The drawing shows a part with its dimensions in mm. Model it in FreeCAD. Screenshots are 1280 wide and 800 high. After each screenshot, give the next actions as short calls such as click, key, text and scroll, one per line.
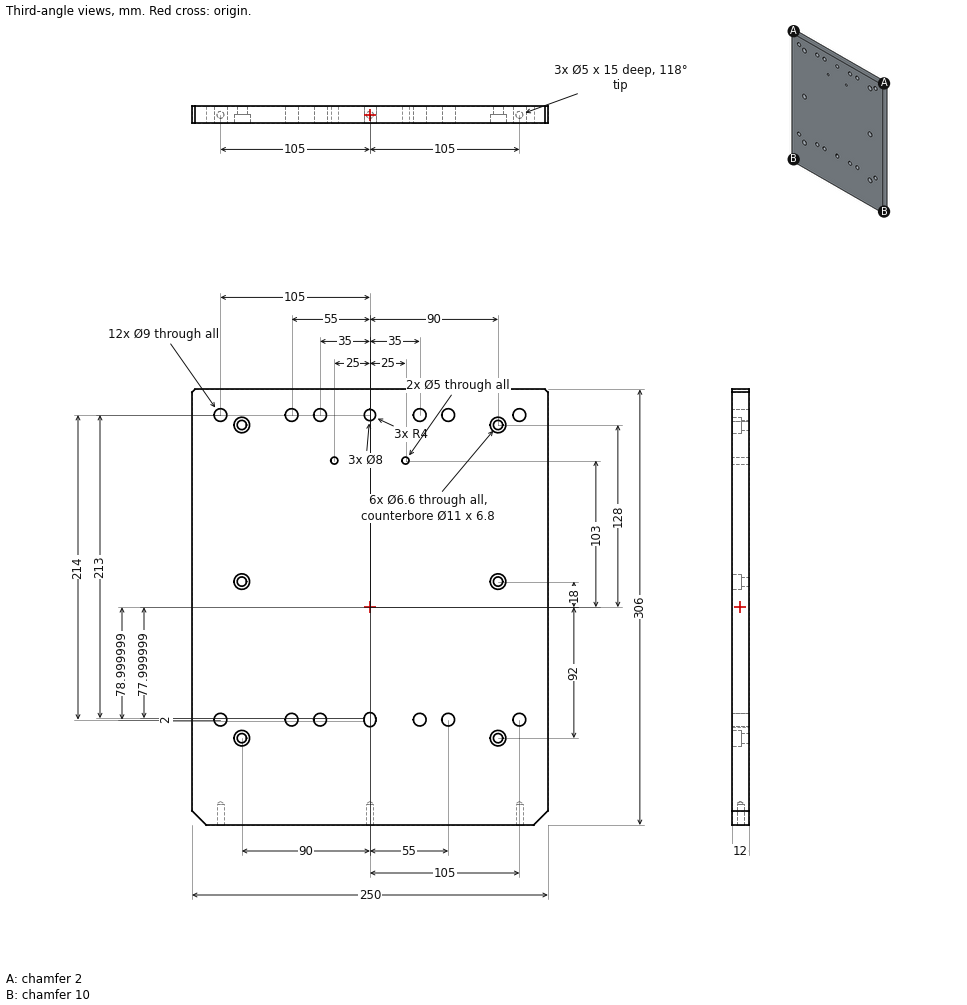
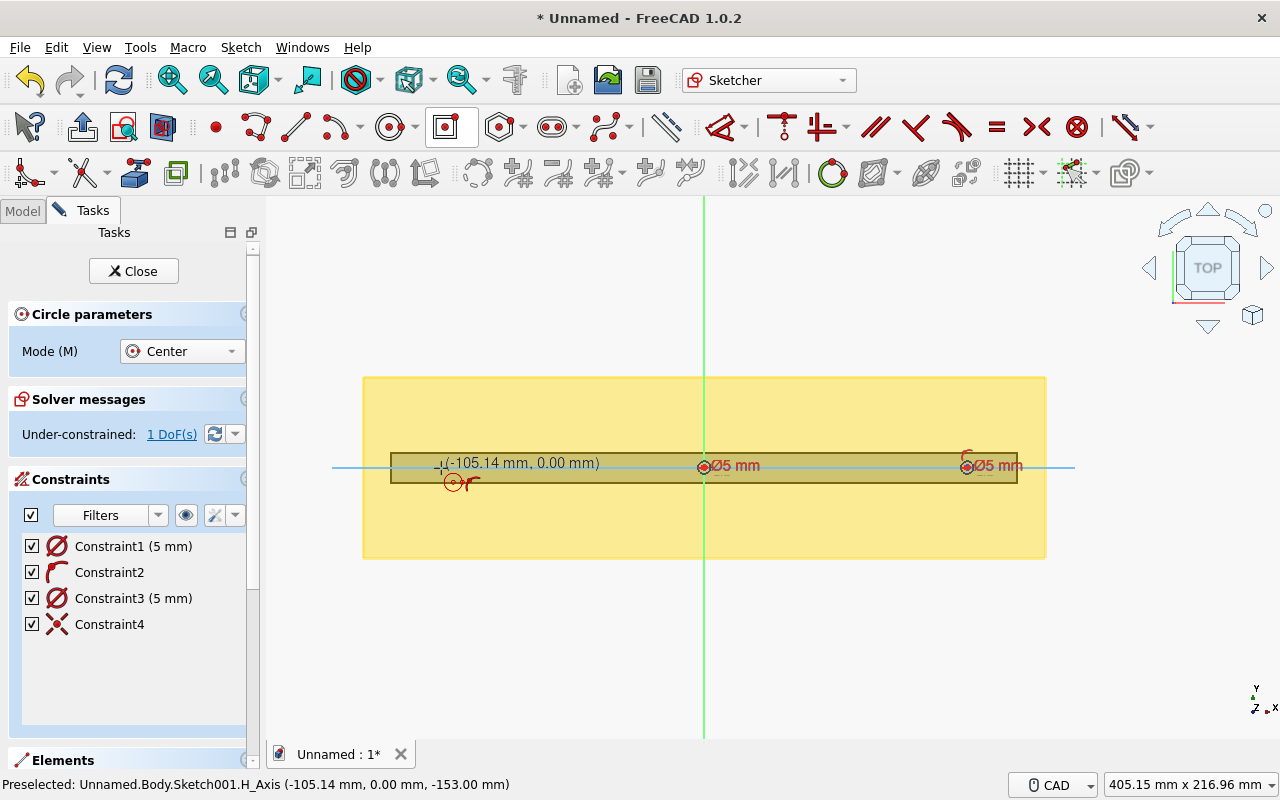
click(441, 468)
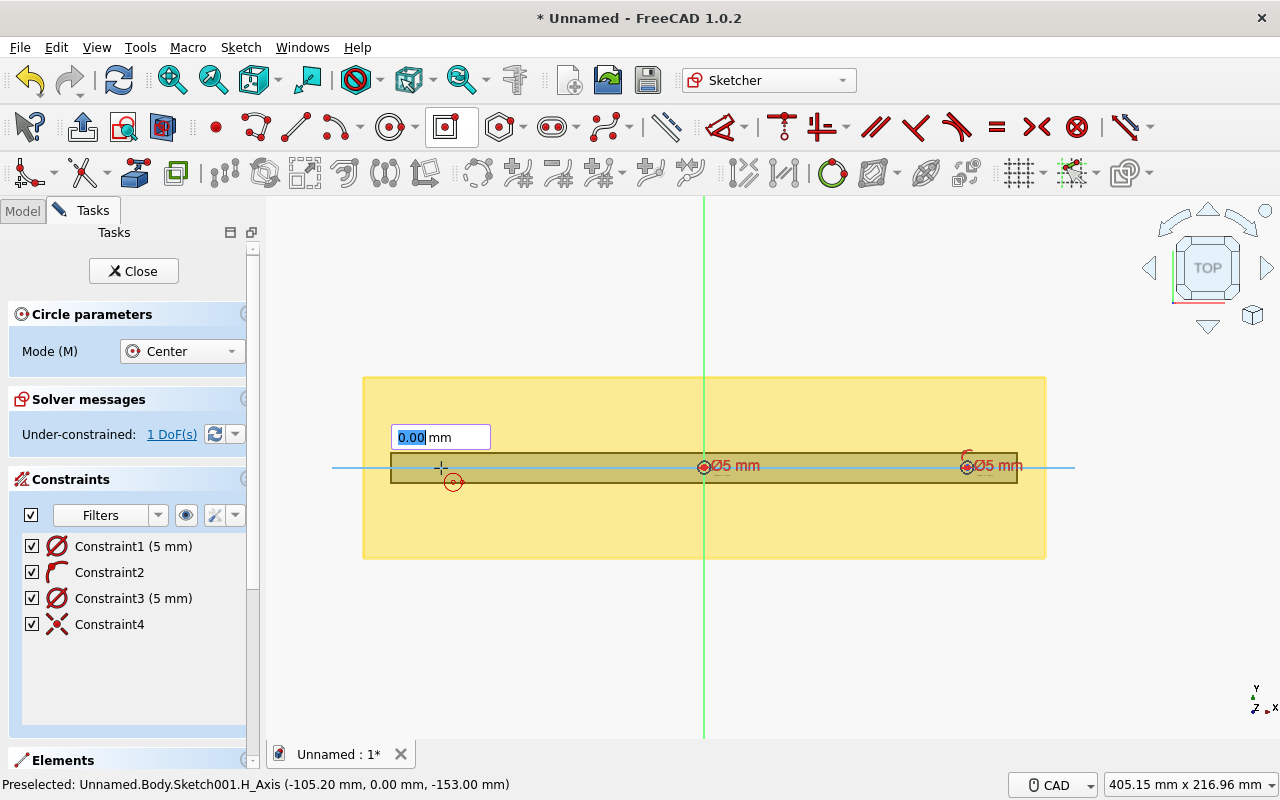
scroll(439, 474, up, 5)
move(440, 472)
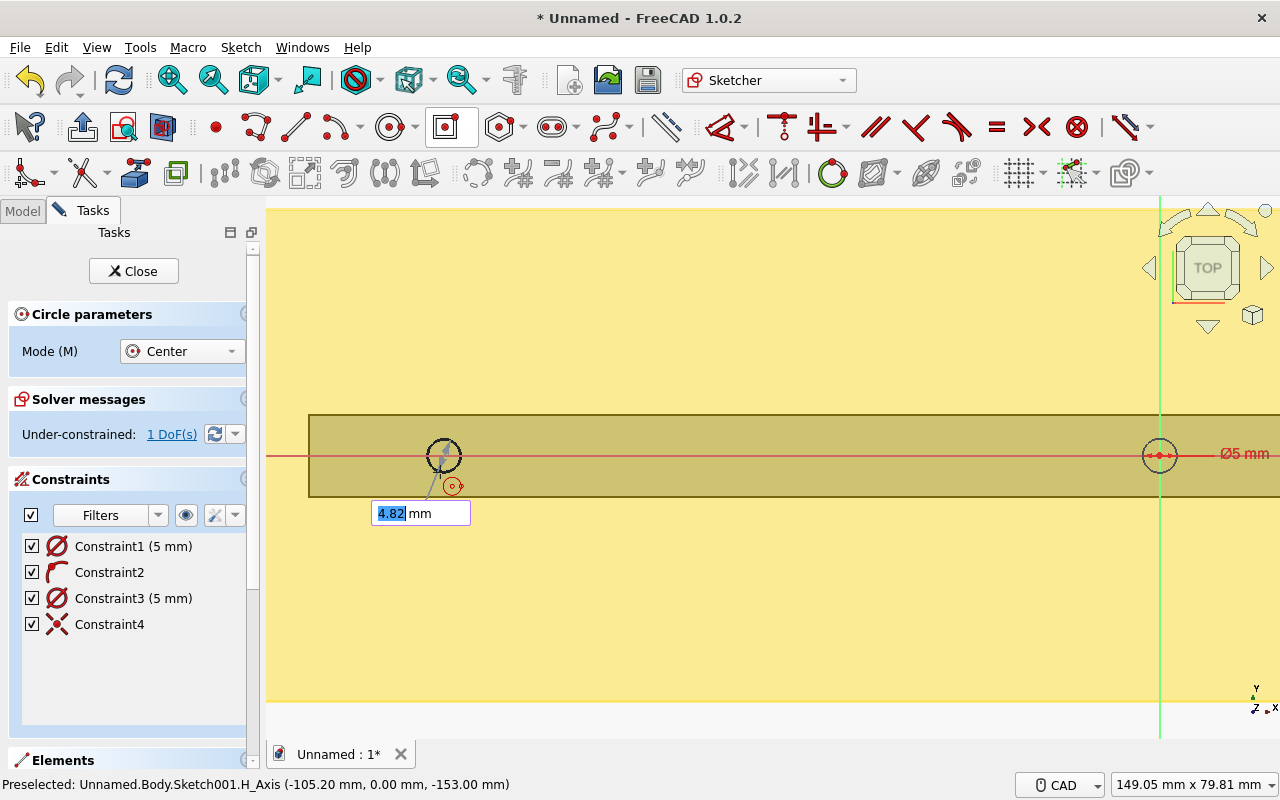
text(5)
key(Return)
key(Escape)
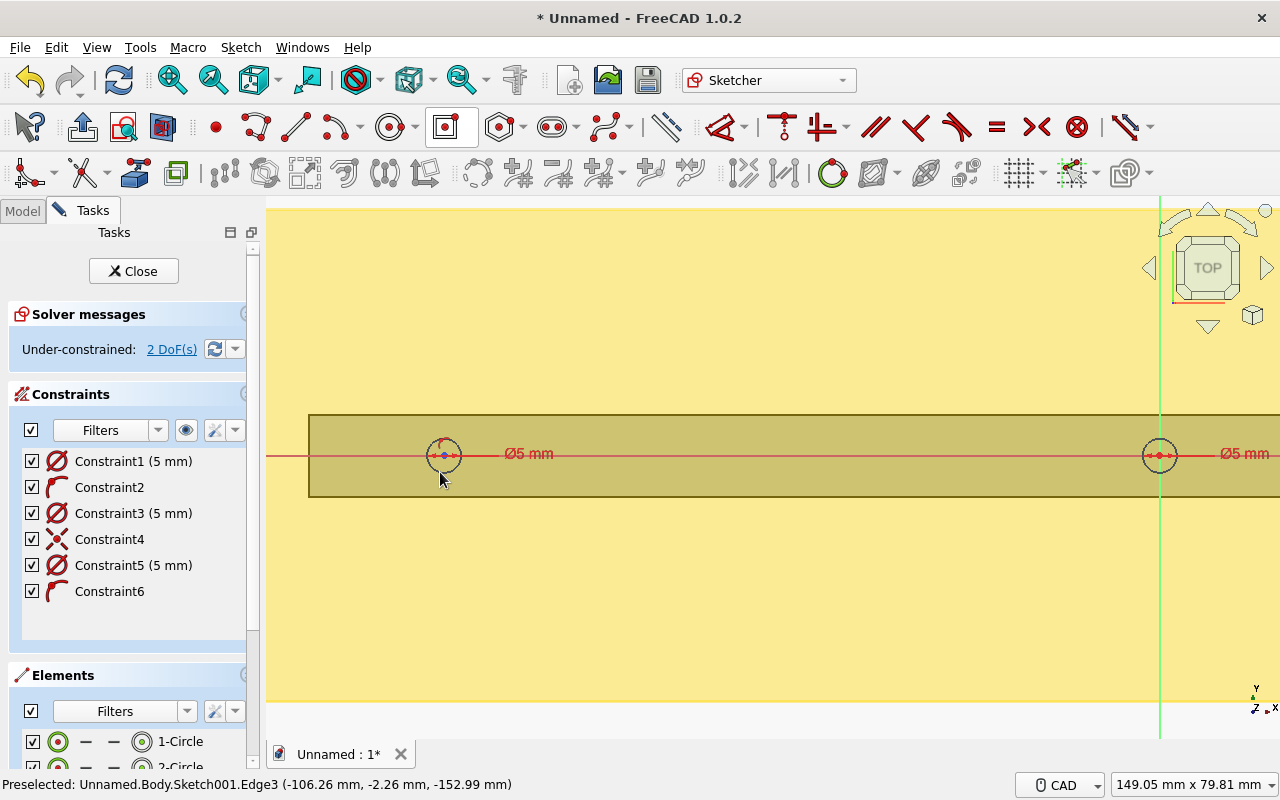
click(720, 128)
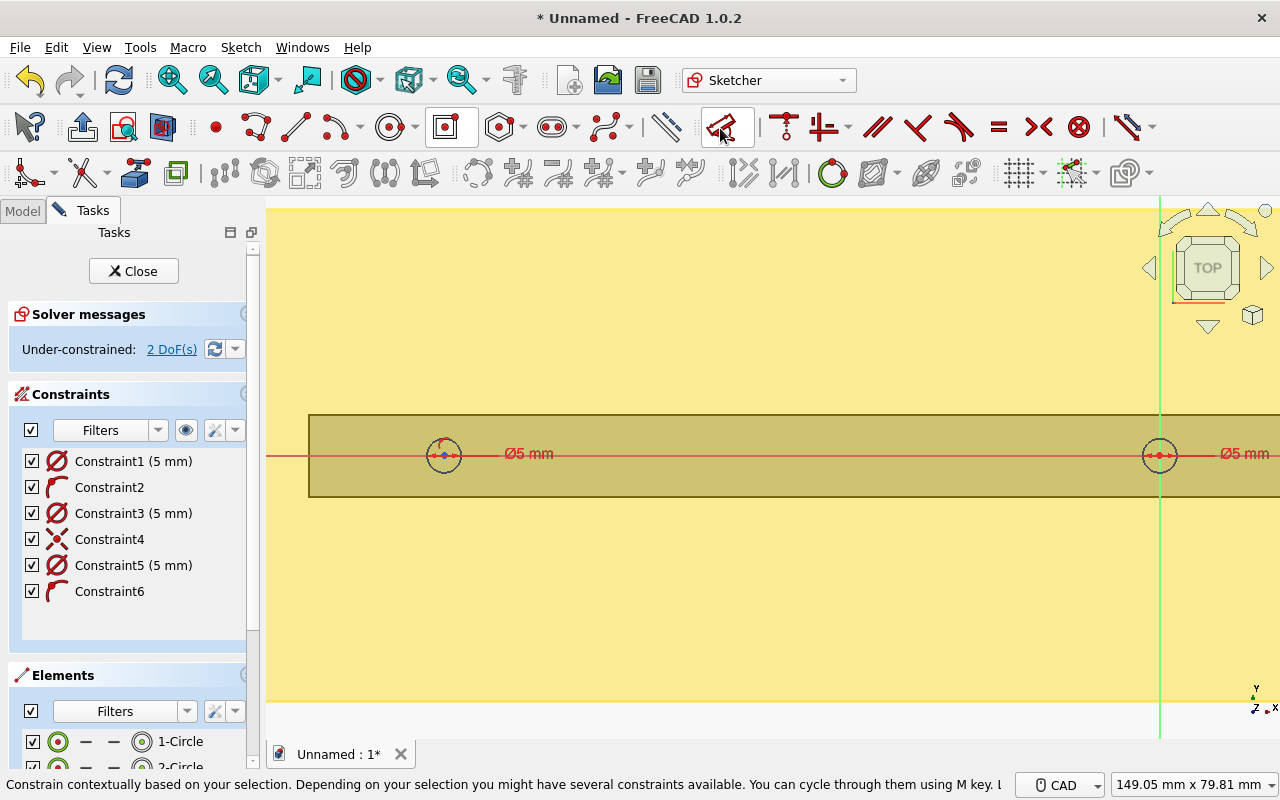
scroll(440, 474, down, 5)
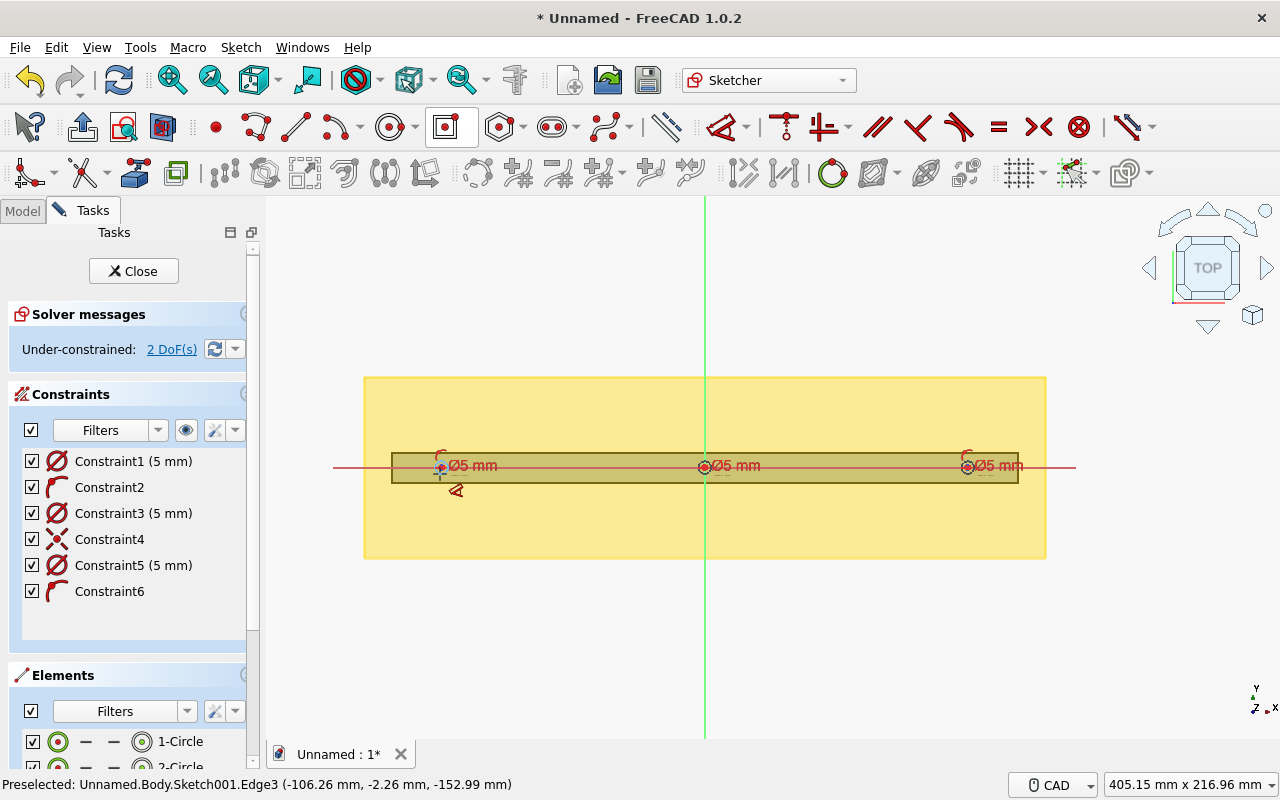
click(968, 468)
click(836, 502)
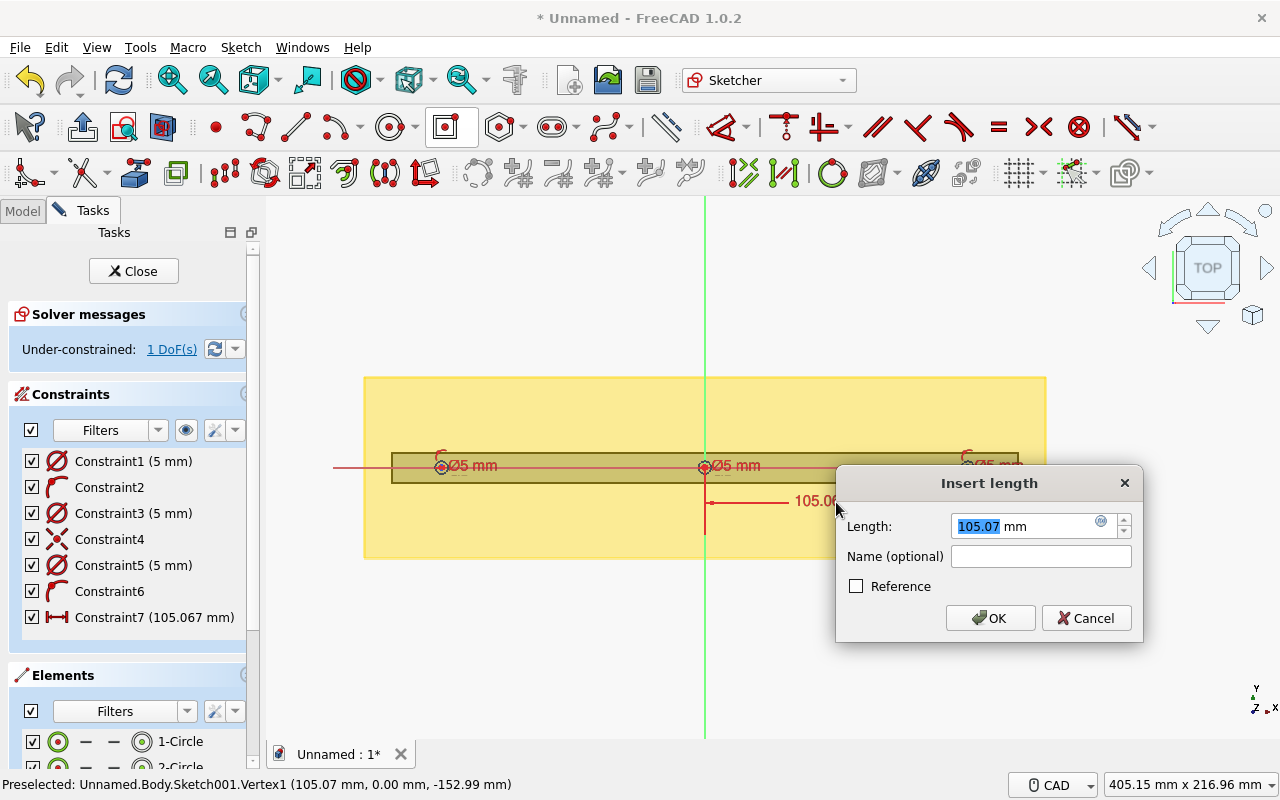
text(105)
key(Return)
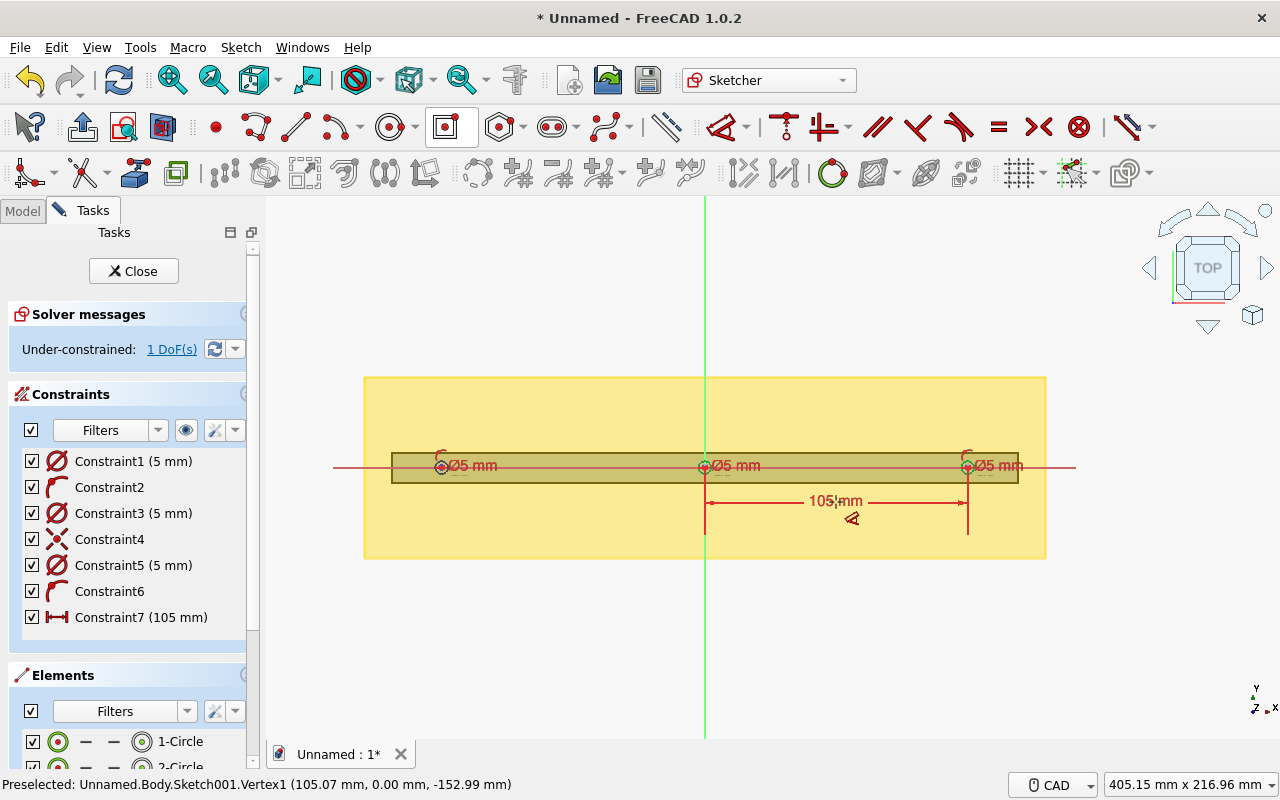
click(442, 468)
click(573, 502)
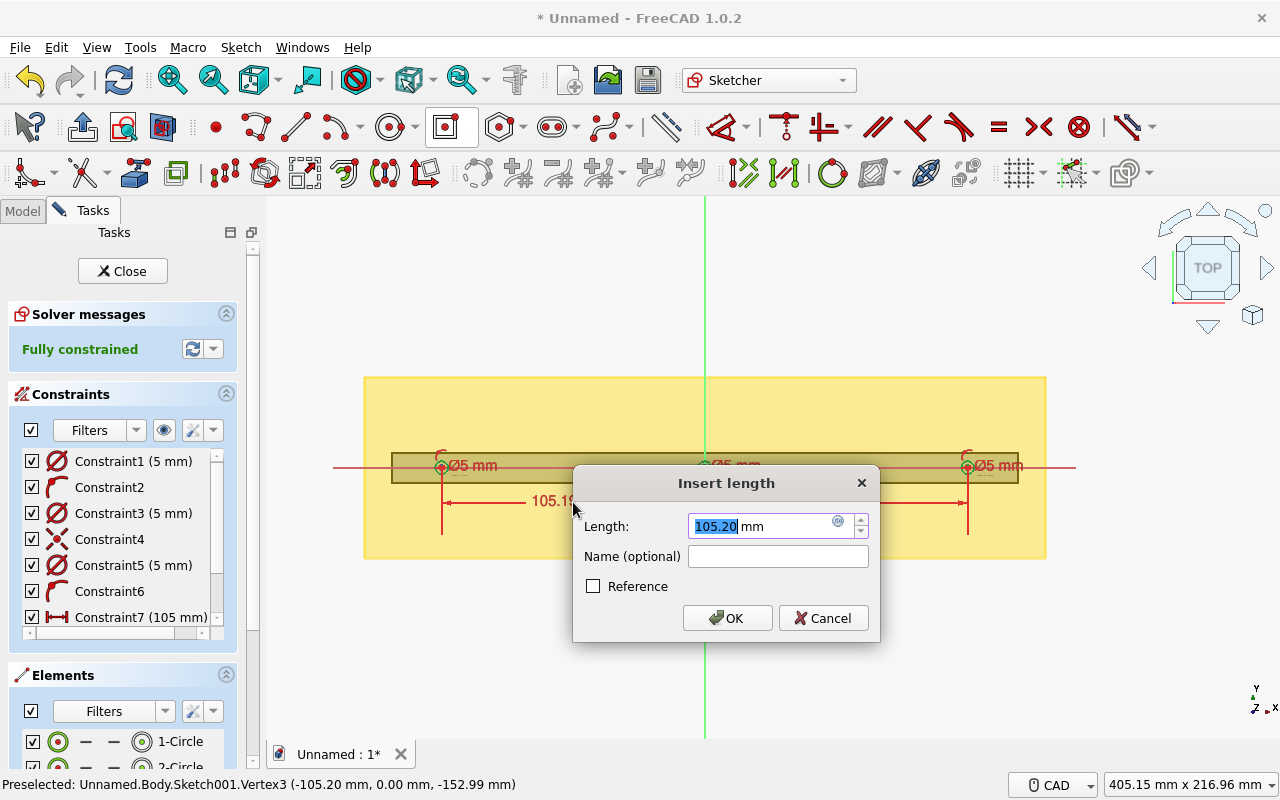
text(105)
key(Return)
key(Escape)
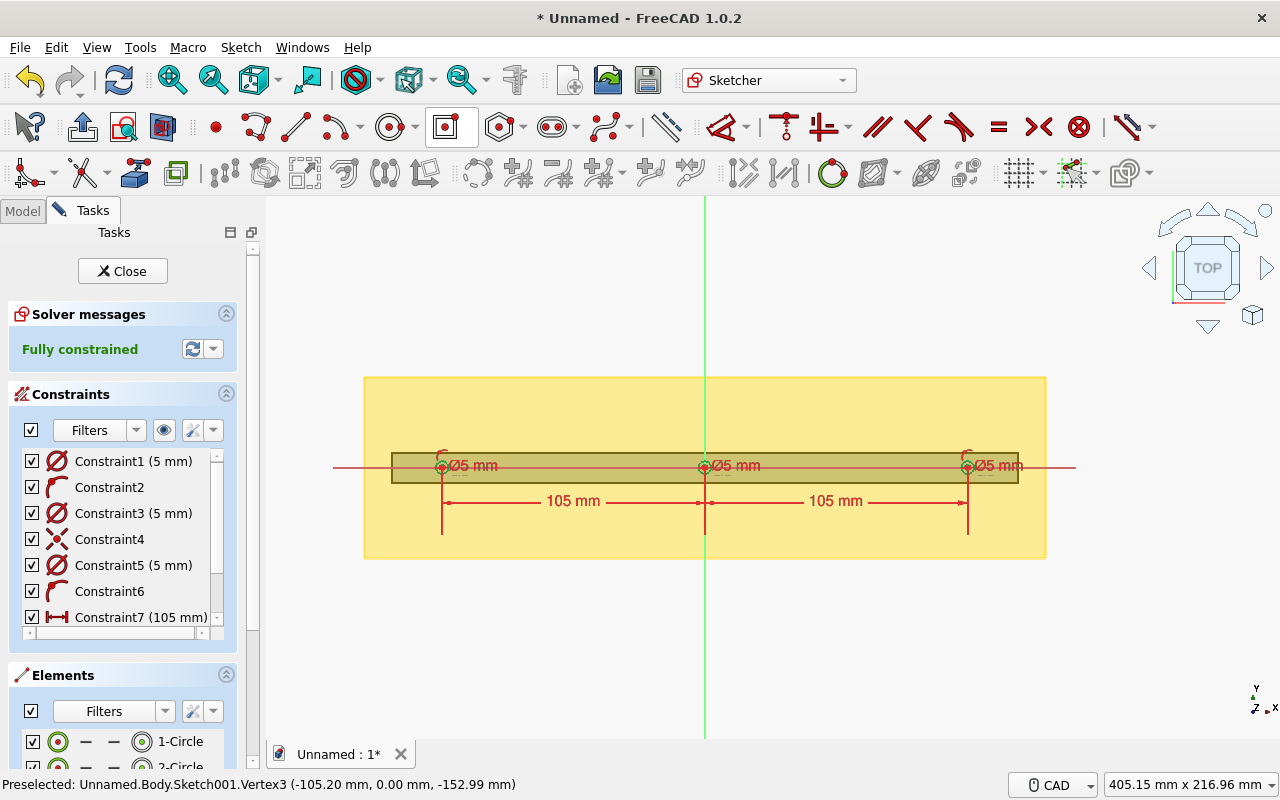
click(123, 271)